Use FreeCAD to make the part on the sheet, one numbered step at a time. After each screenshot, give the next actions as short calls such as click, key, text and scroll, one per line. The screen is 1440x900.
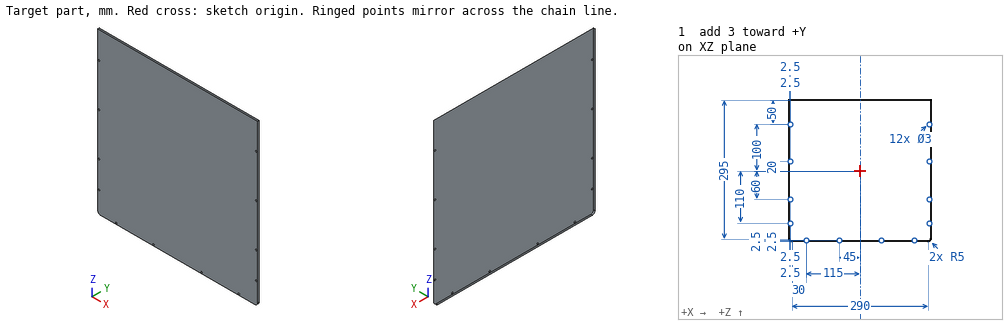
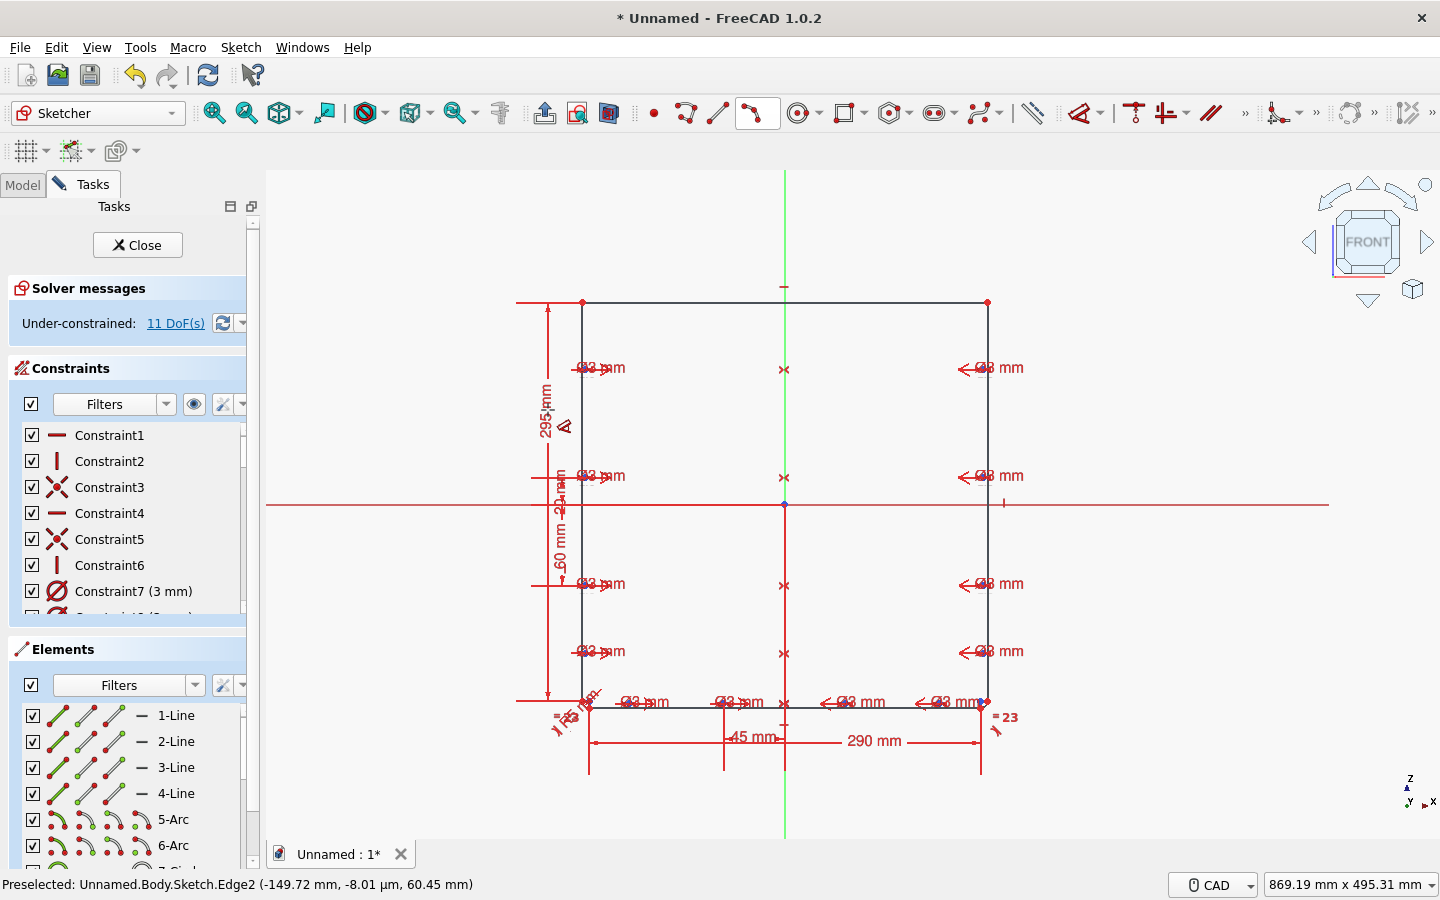
click(585, 370)
click(551, 437)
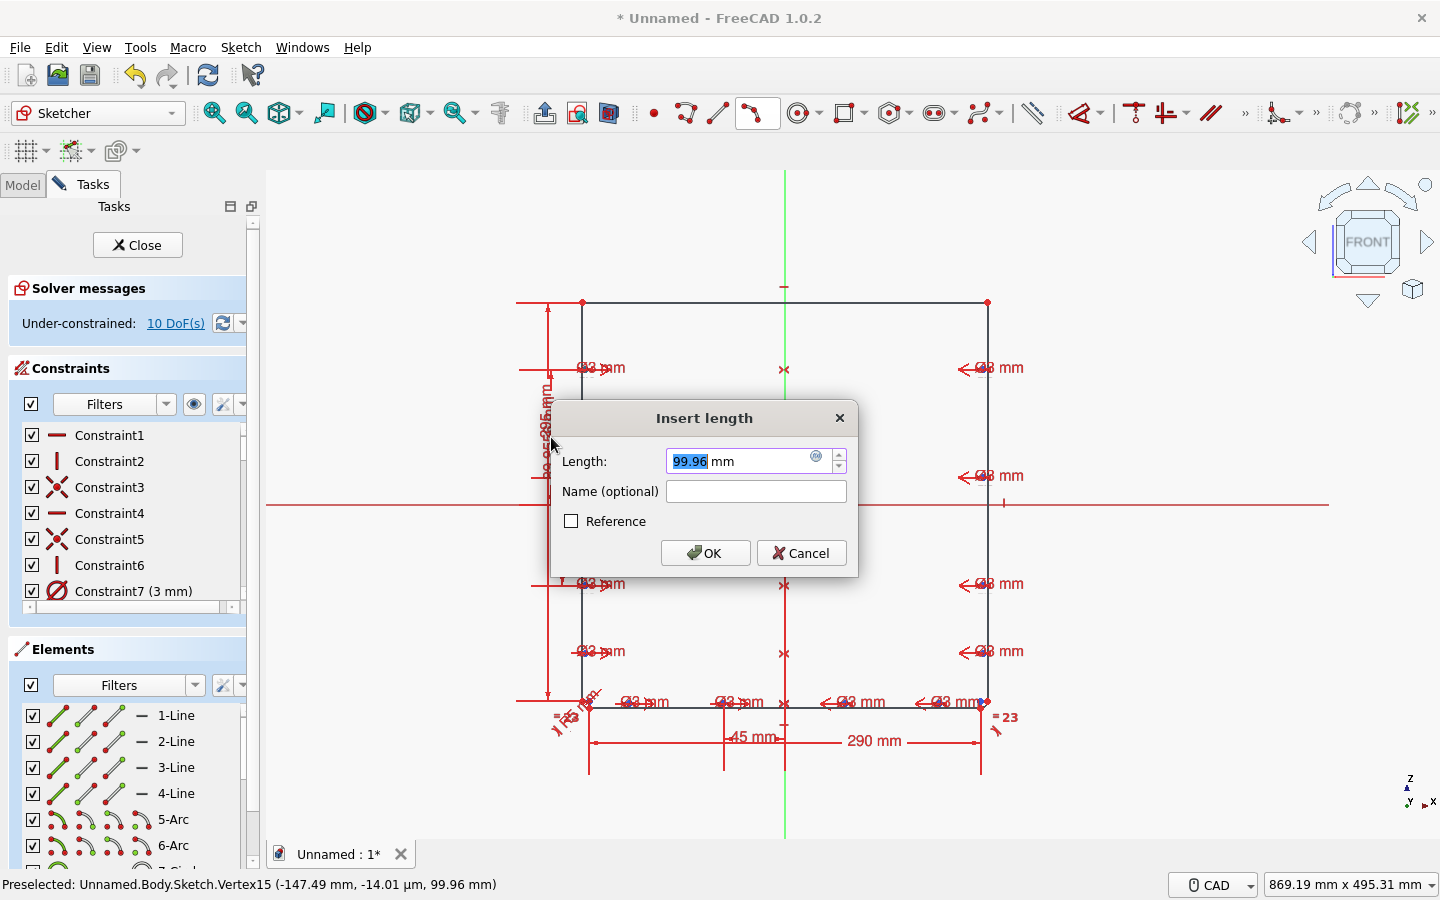
text(100)
key(Return)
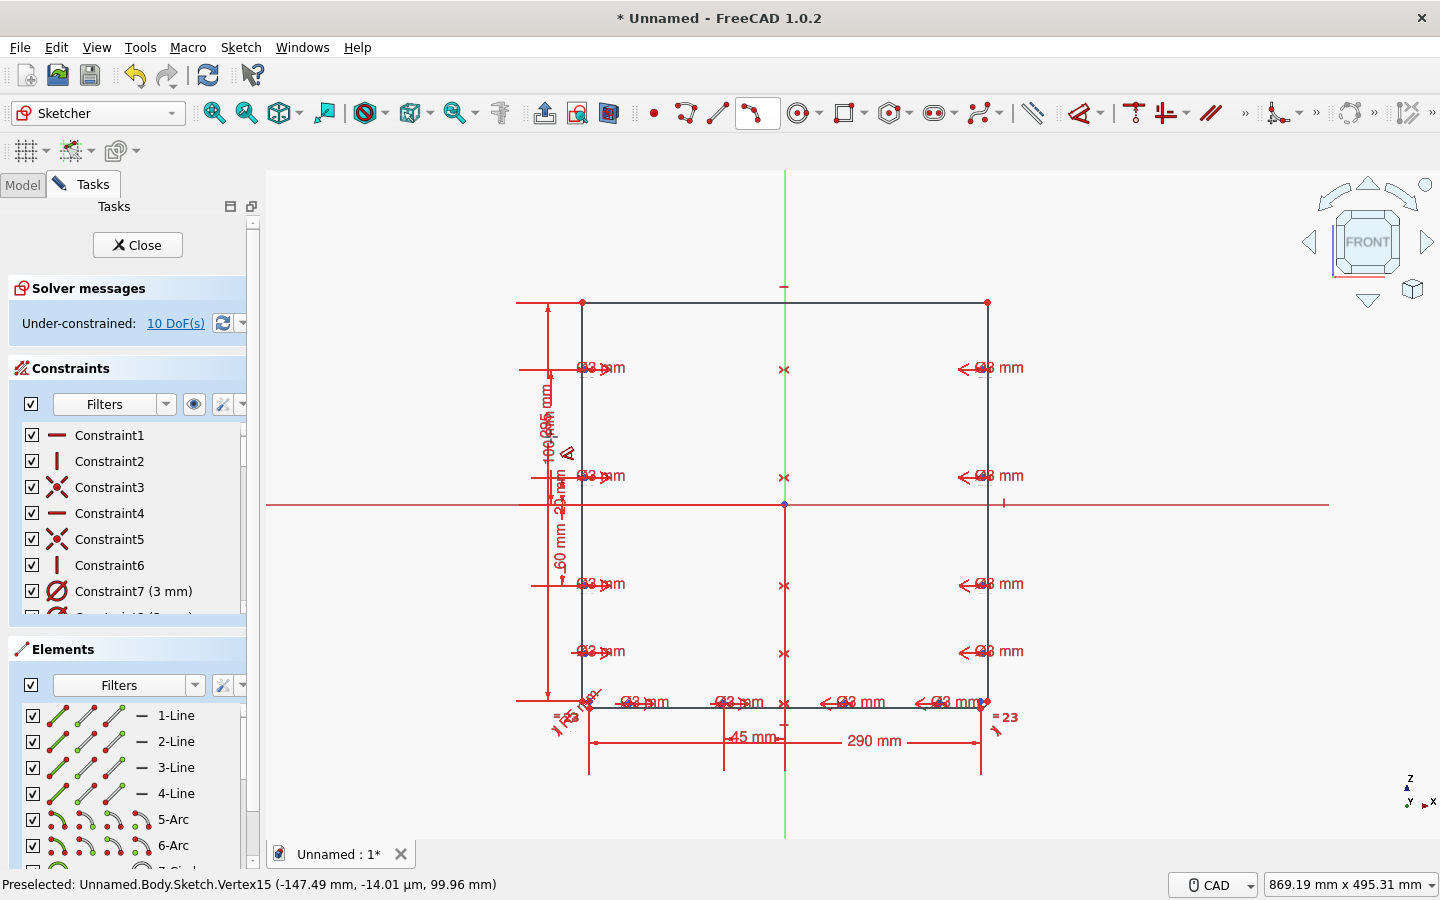
click(585, 653)
click(551, 579)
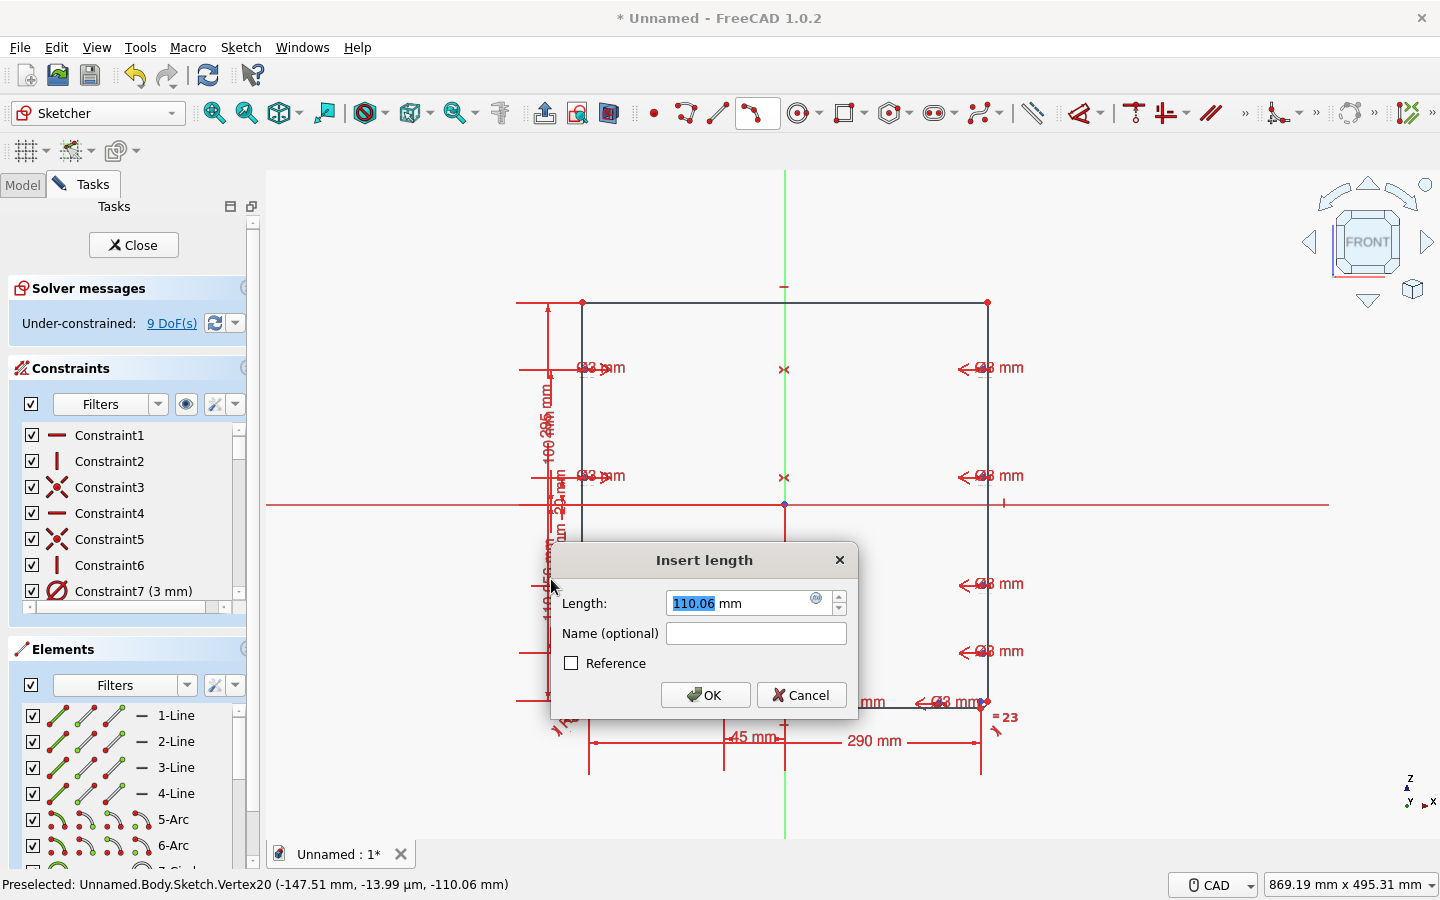
text(110)
key(Return)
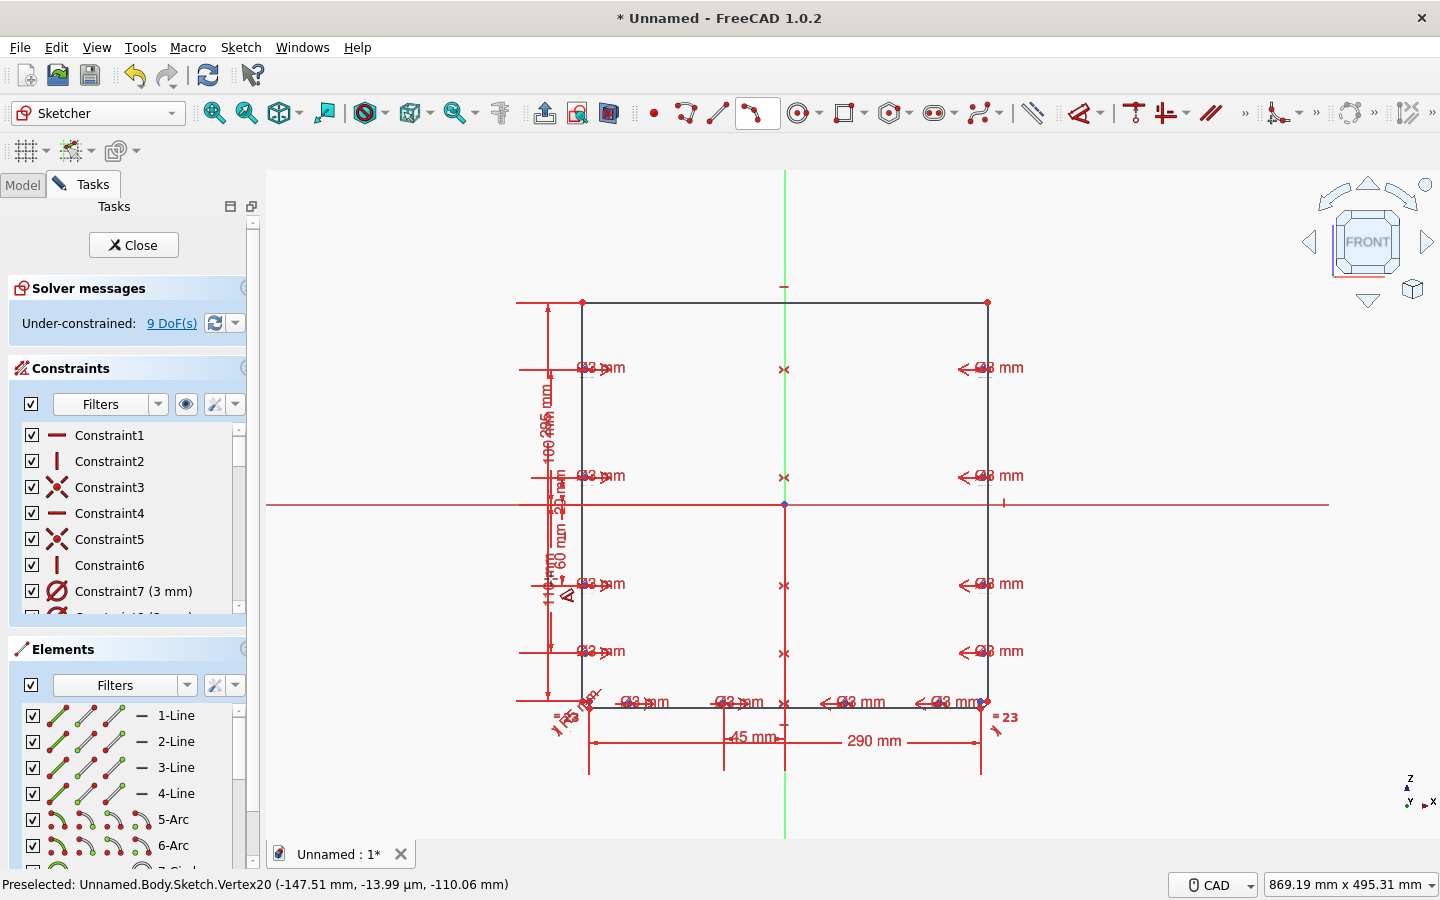
click(629, 704)
click(671, 738)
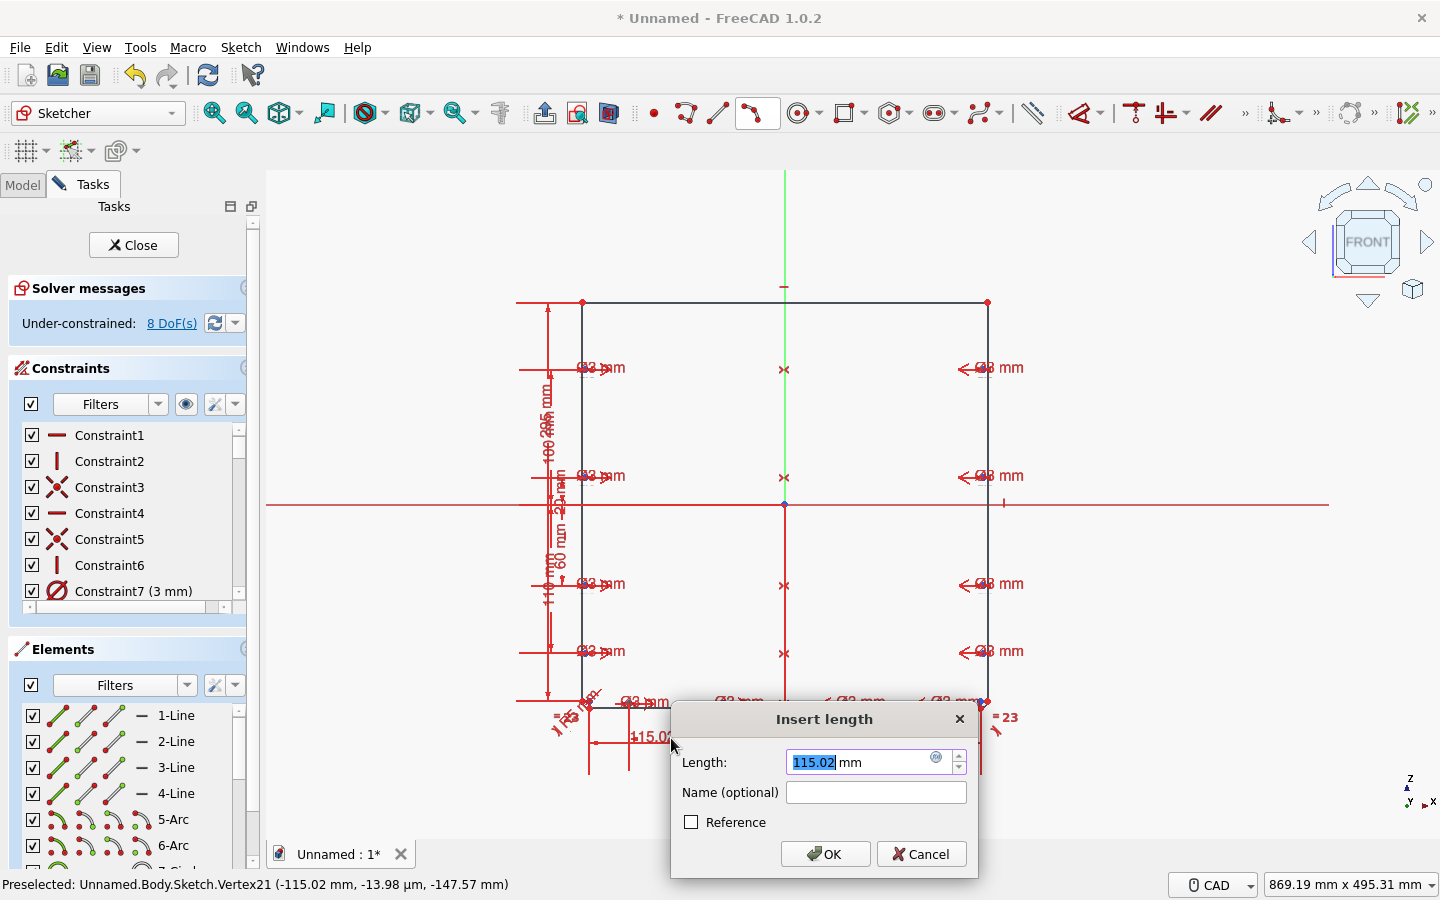
text(115)
key(Return)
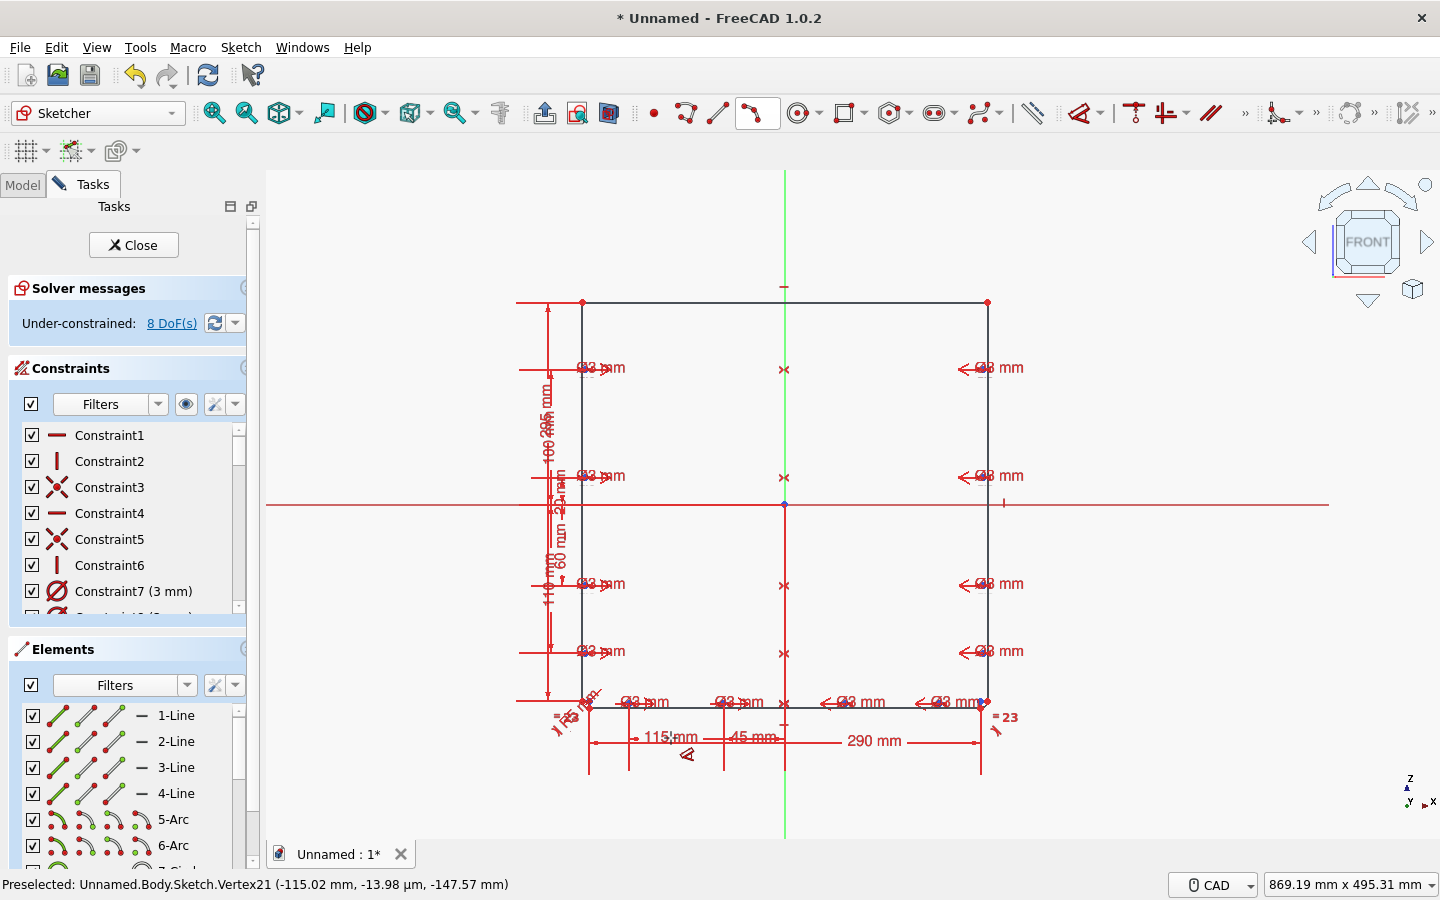
click(582, 303)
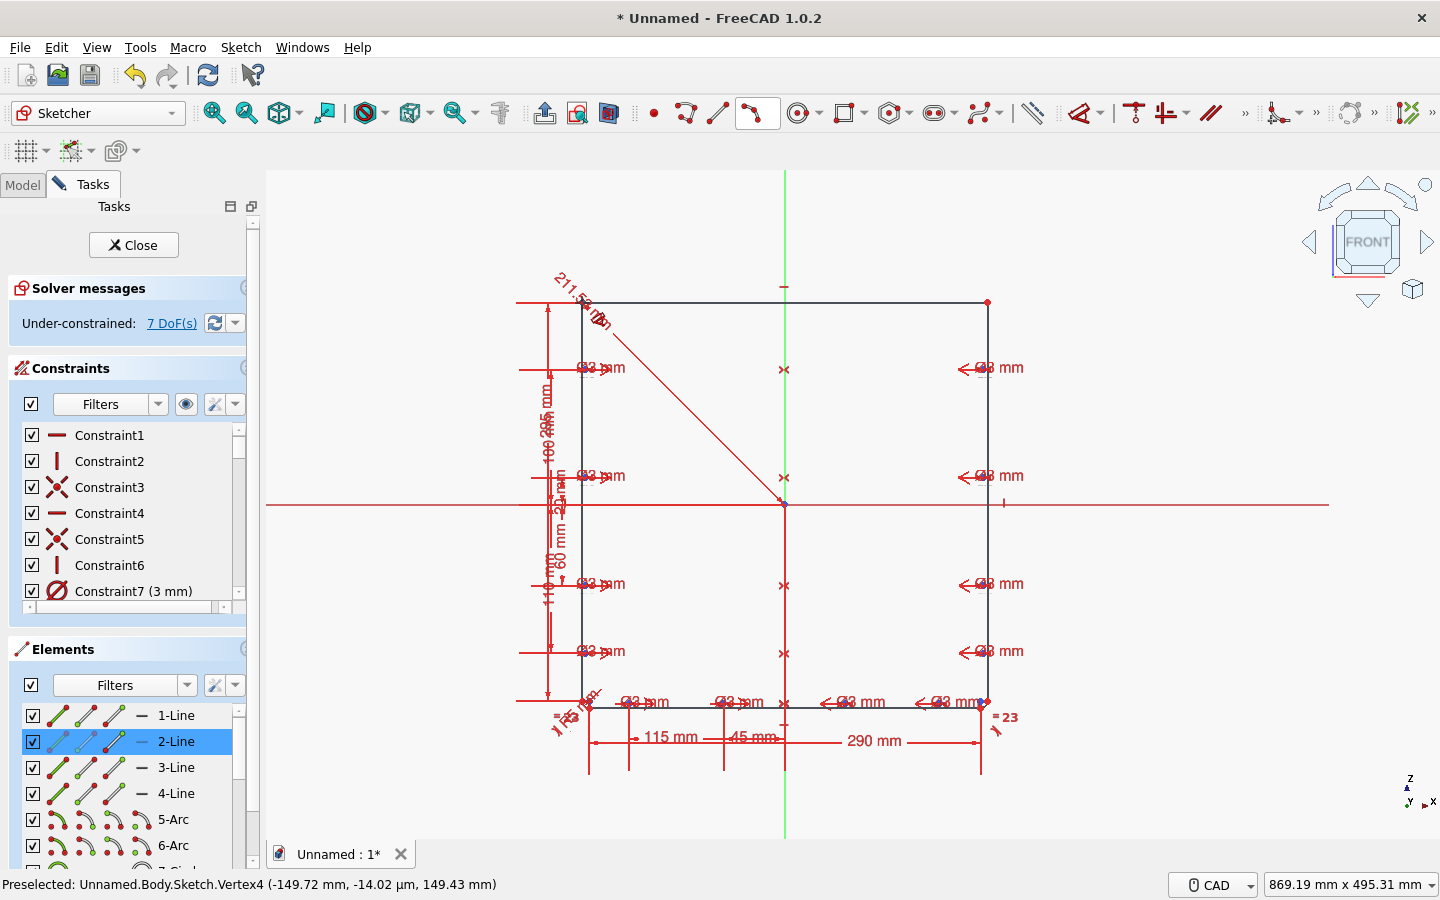
click(585, 370)
click(548, 336)